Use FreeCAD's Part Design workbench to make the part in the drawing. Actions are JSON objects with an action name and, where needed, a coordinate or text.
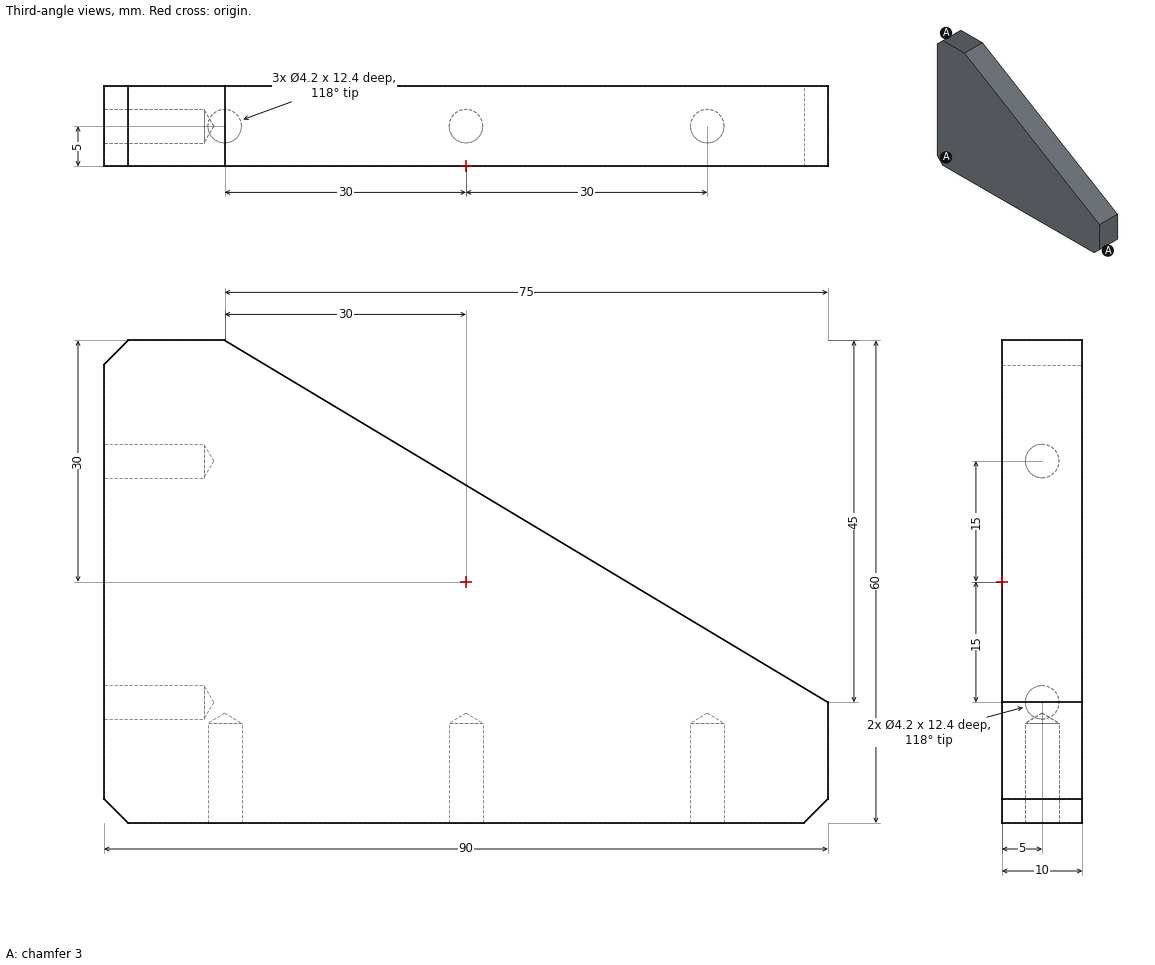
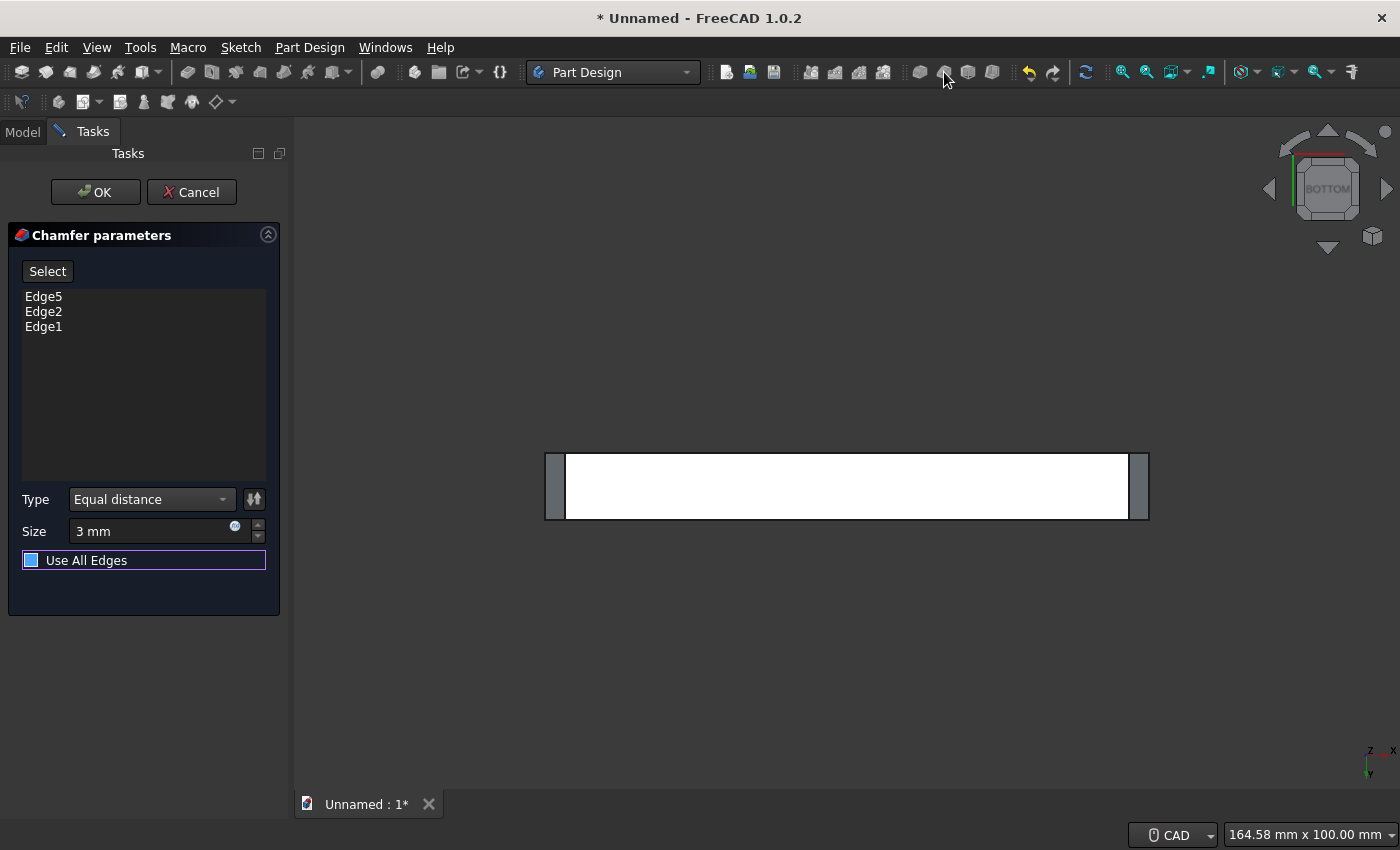
{"action": "left_click", "coordinate": [96, 192]}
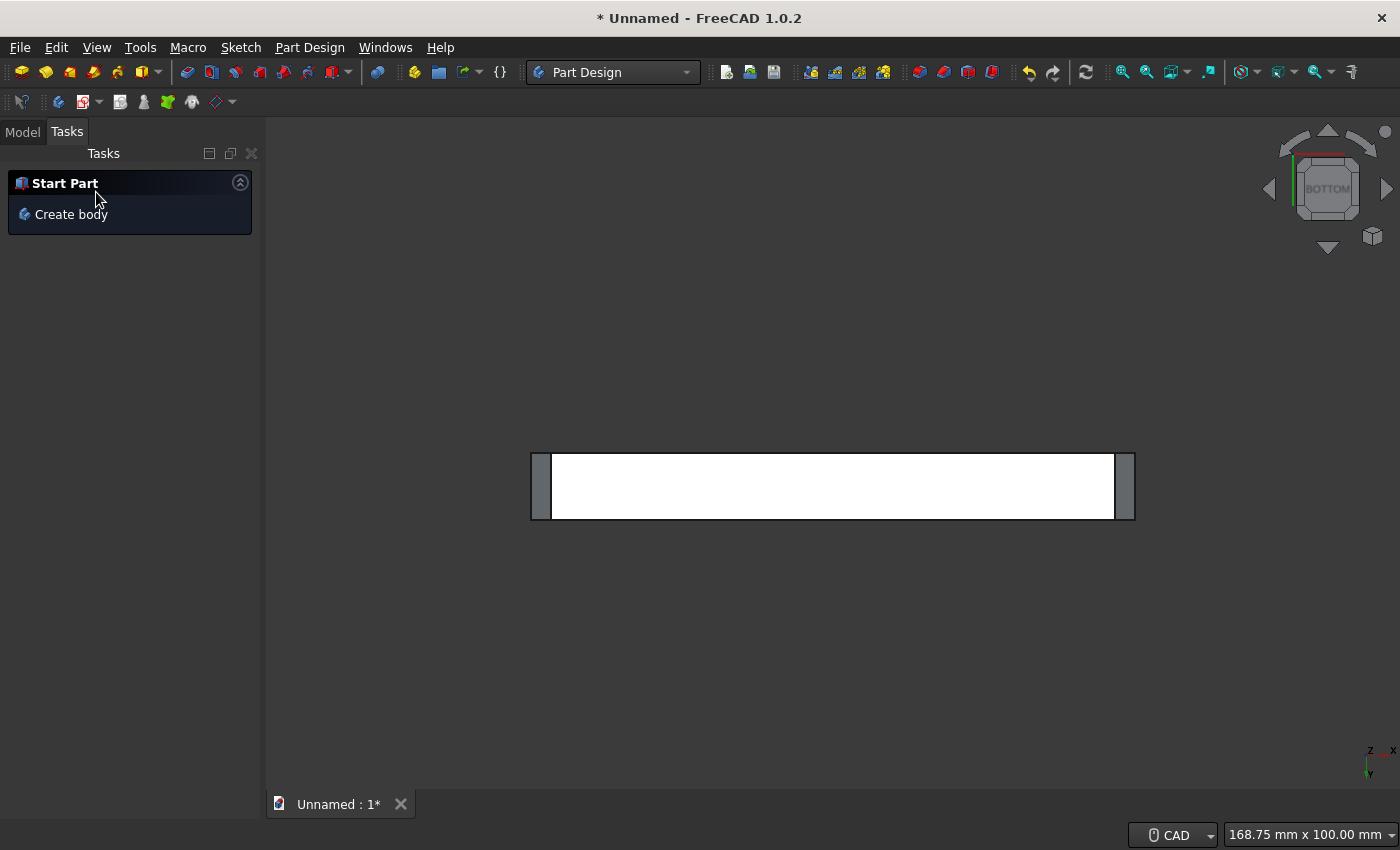
{"action": "key", "text": "6"}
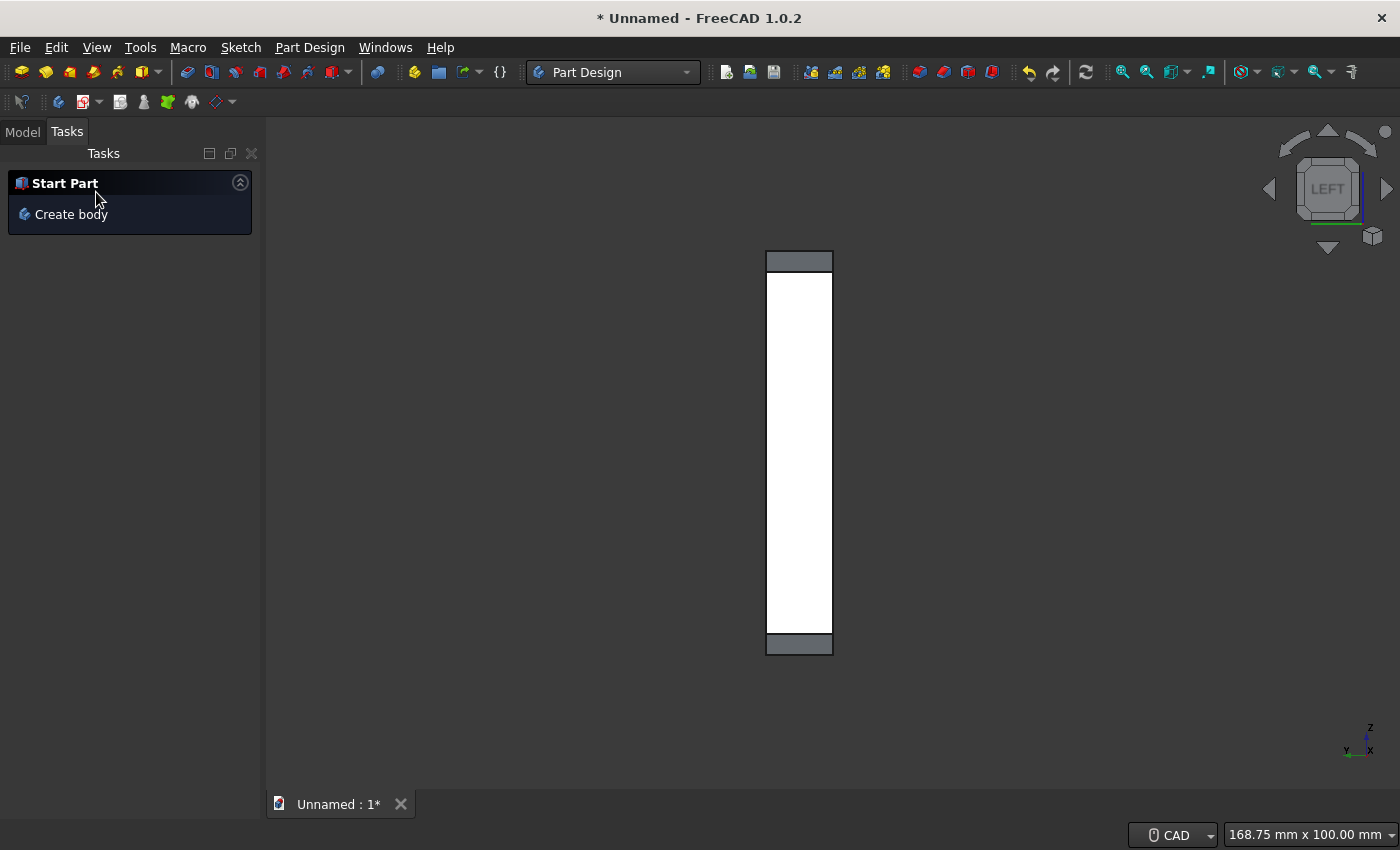
{"action": "left_click", "coordinate": [799, 504]}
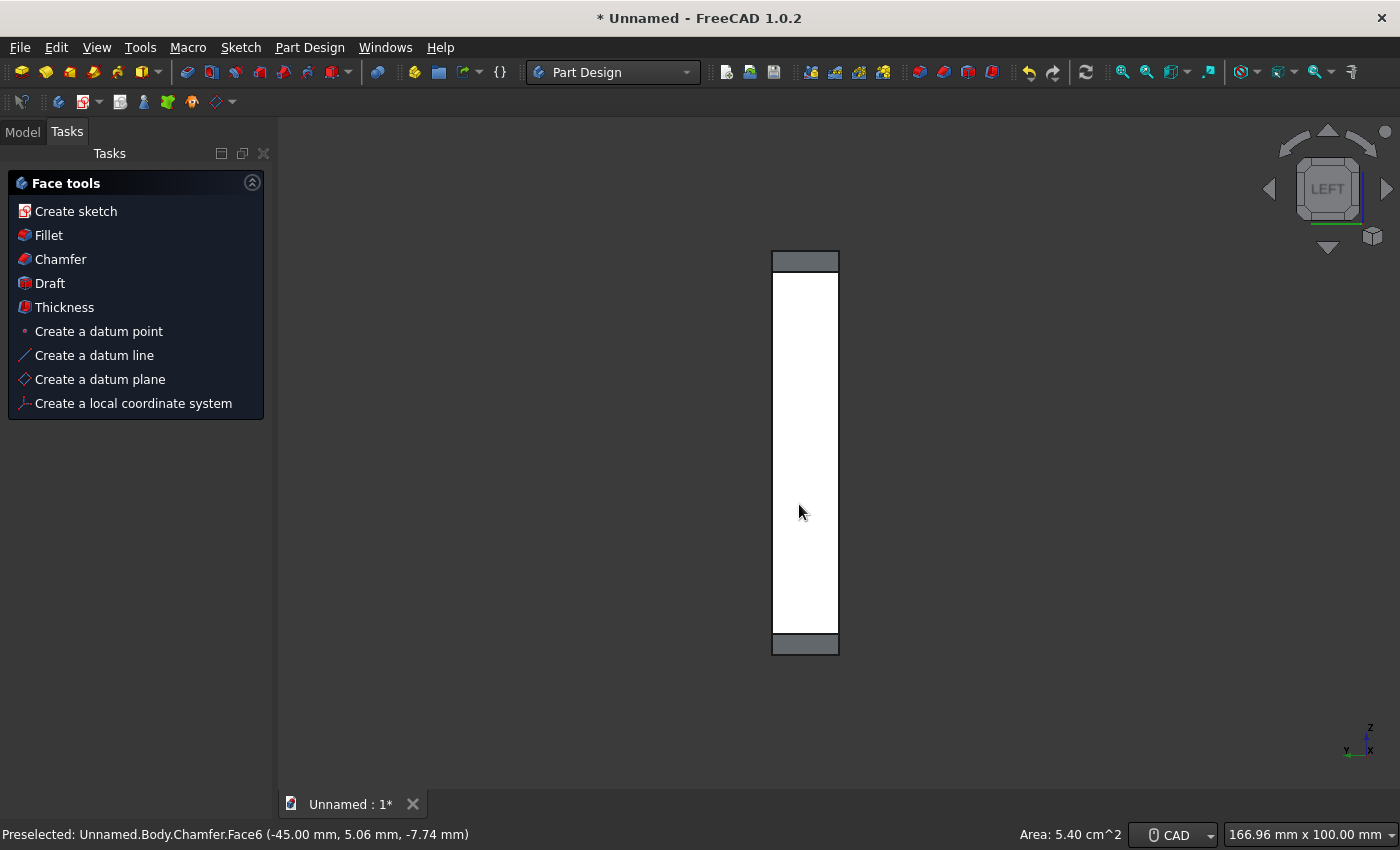
{"action": "left_click", "coordinate": [84, 102]}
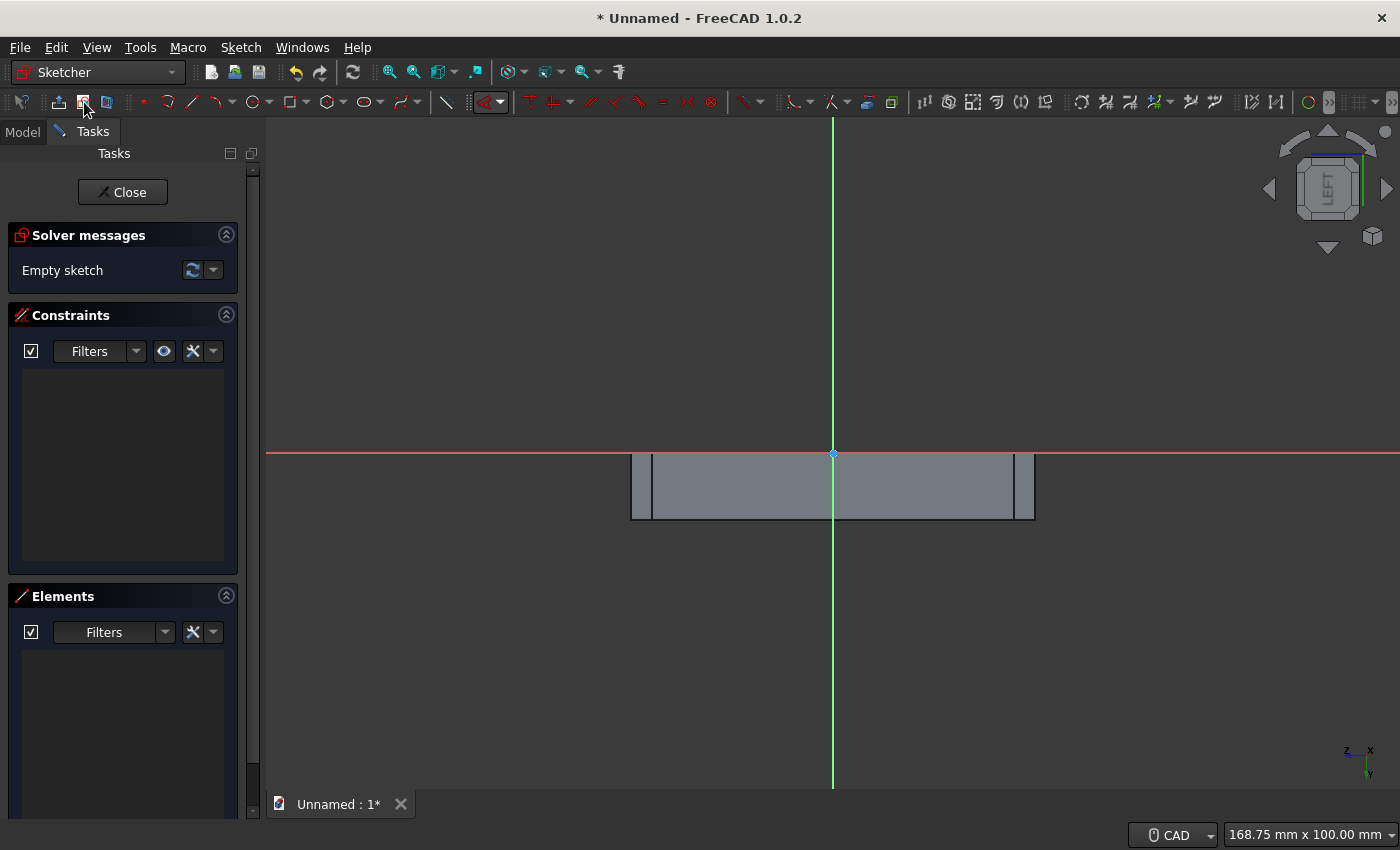
{"action": "scroll", "coordinate": [873, 491], "scroll_direction": "up", "scroll_amount": 5}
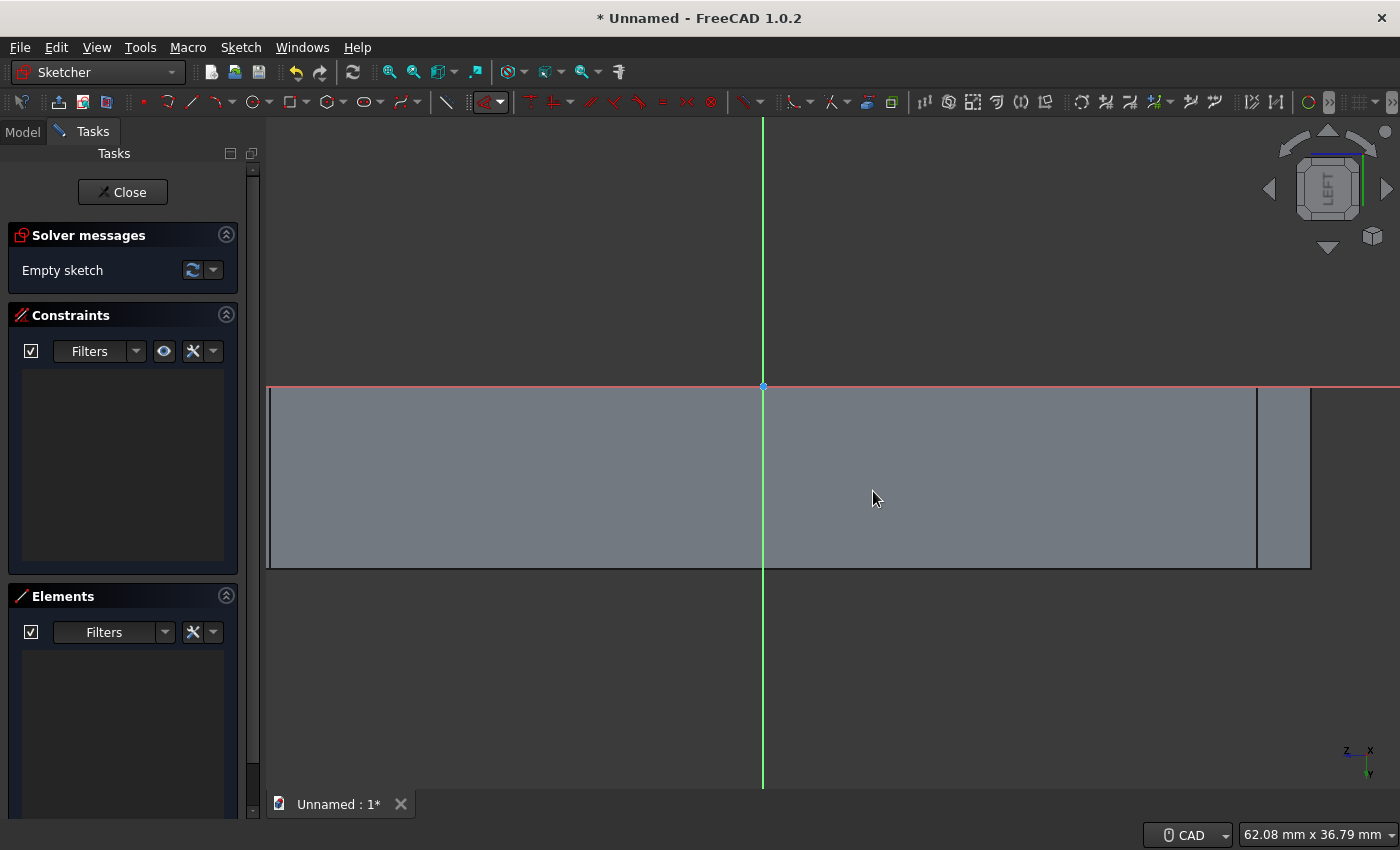
{"action": "left_click", "coordinate": [254, 102]}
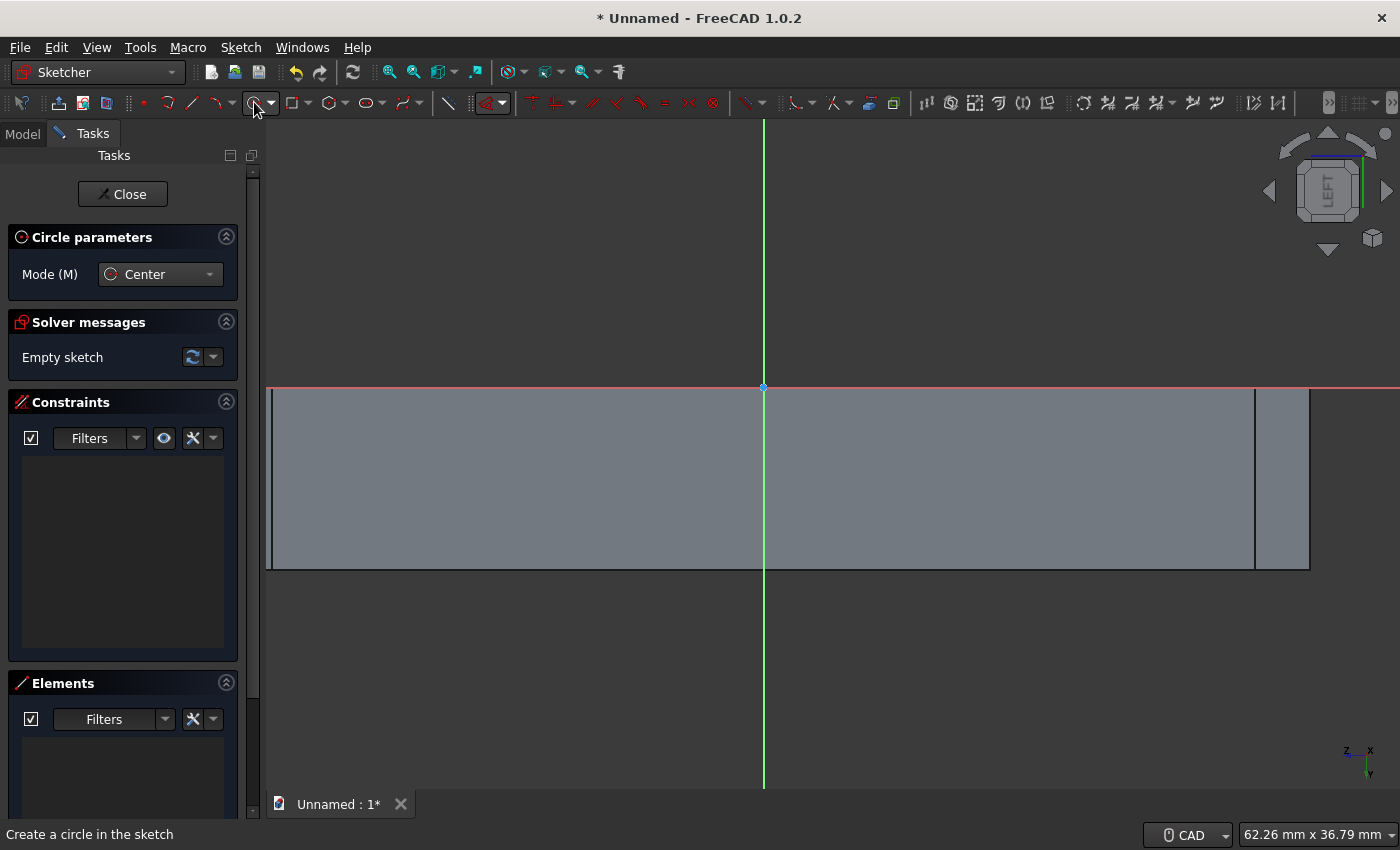
{"action": "left_click", "coordinate": [1037, 479]}
{"action": "mouse_move", "coordinate": [1064, 452]}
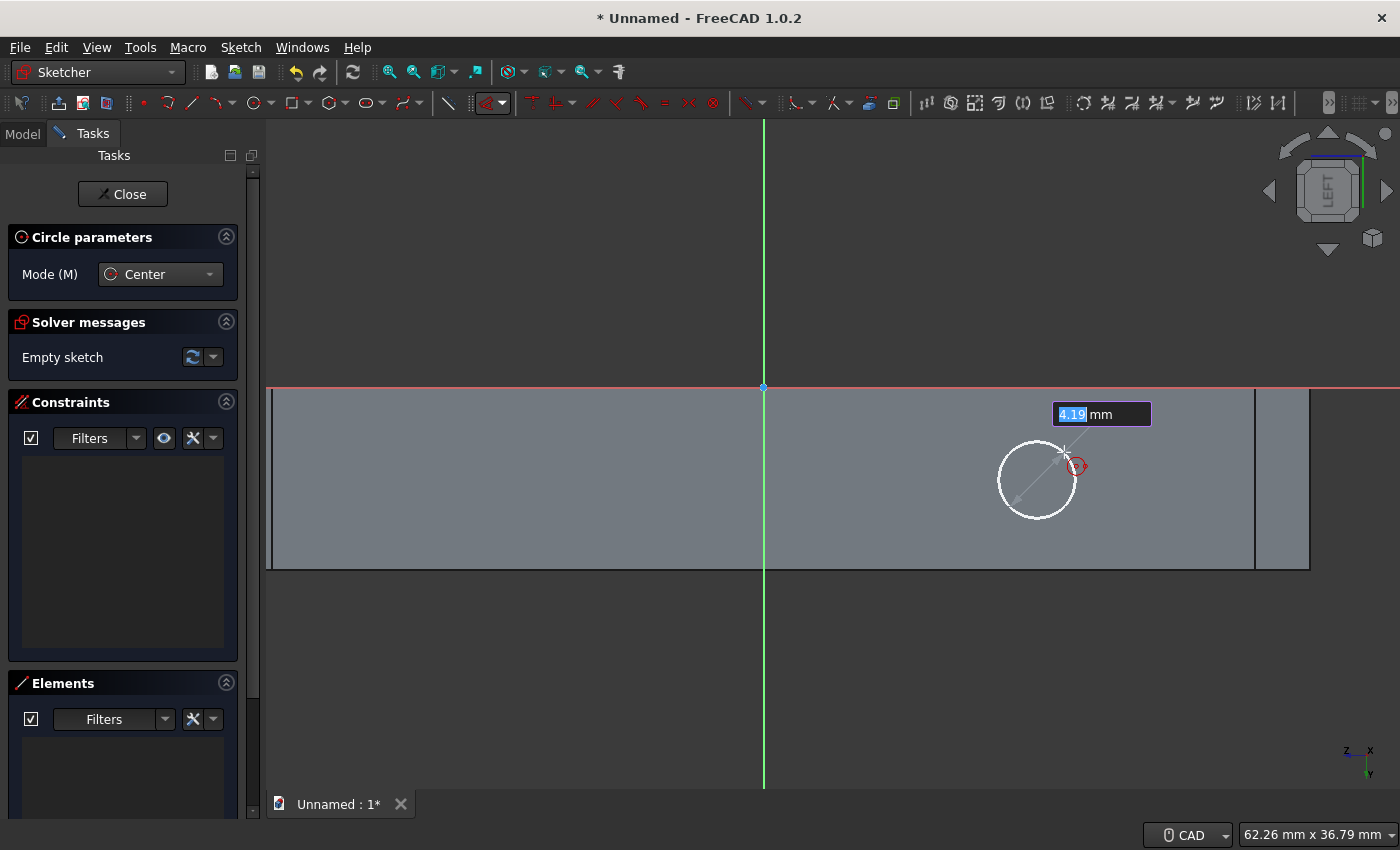
{"action": "type", "text": "4.2"}
{"action": "key", "text": "Return"}